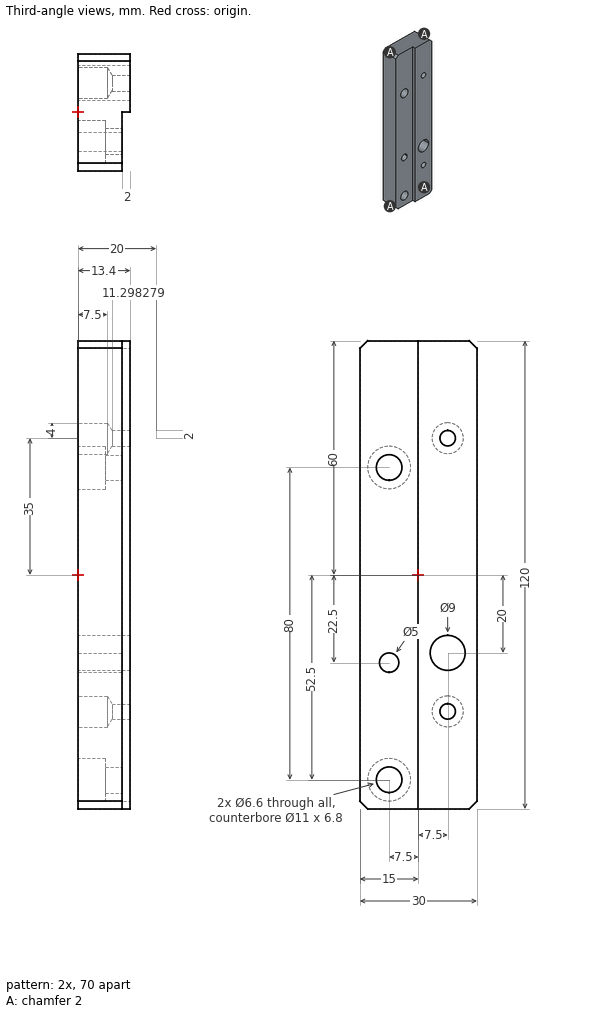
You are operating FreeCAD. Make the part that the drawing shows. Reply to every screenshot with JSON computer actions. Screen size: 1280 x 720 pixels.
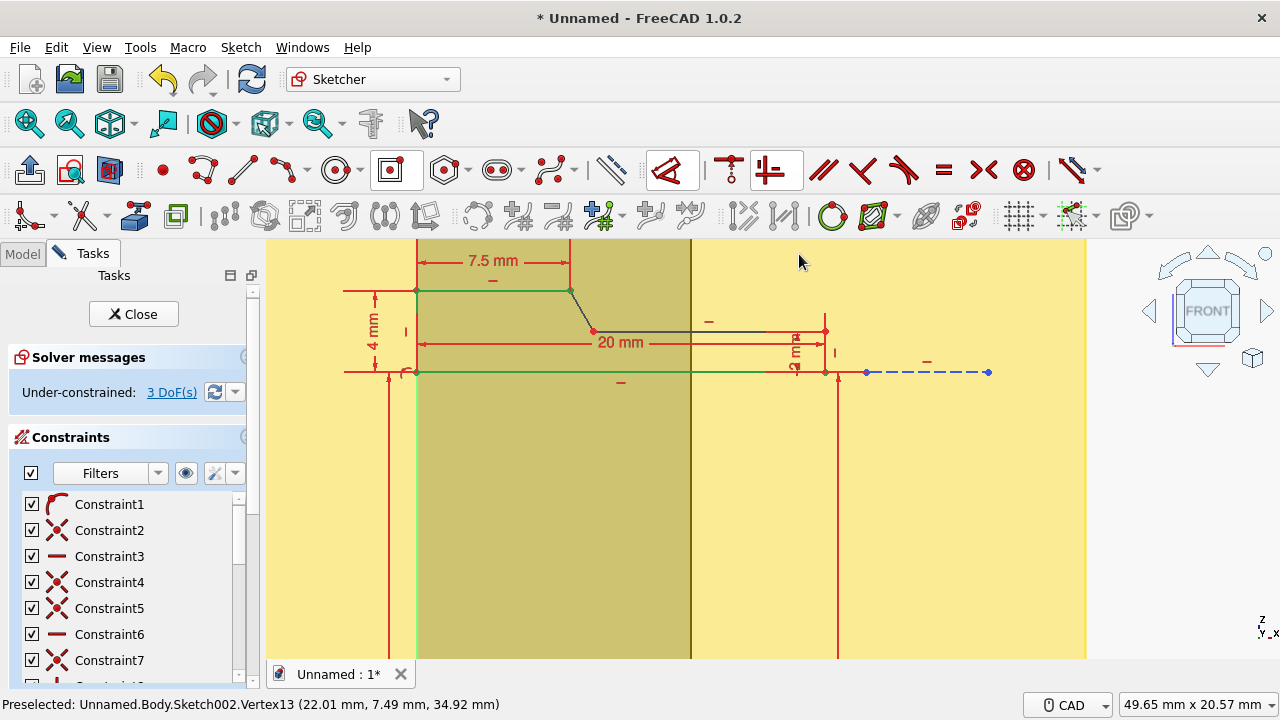
{"action": "left_click", "coordinate": [663, 332]}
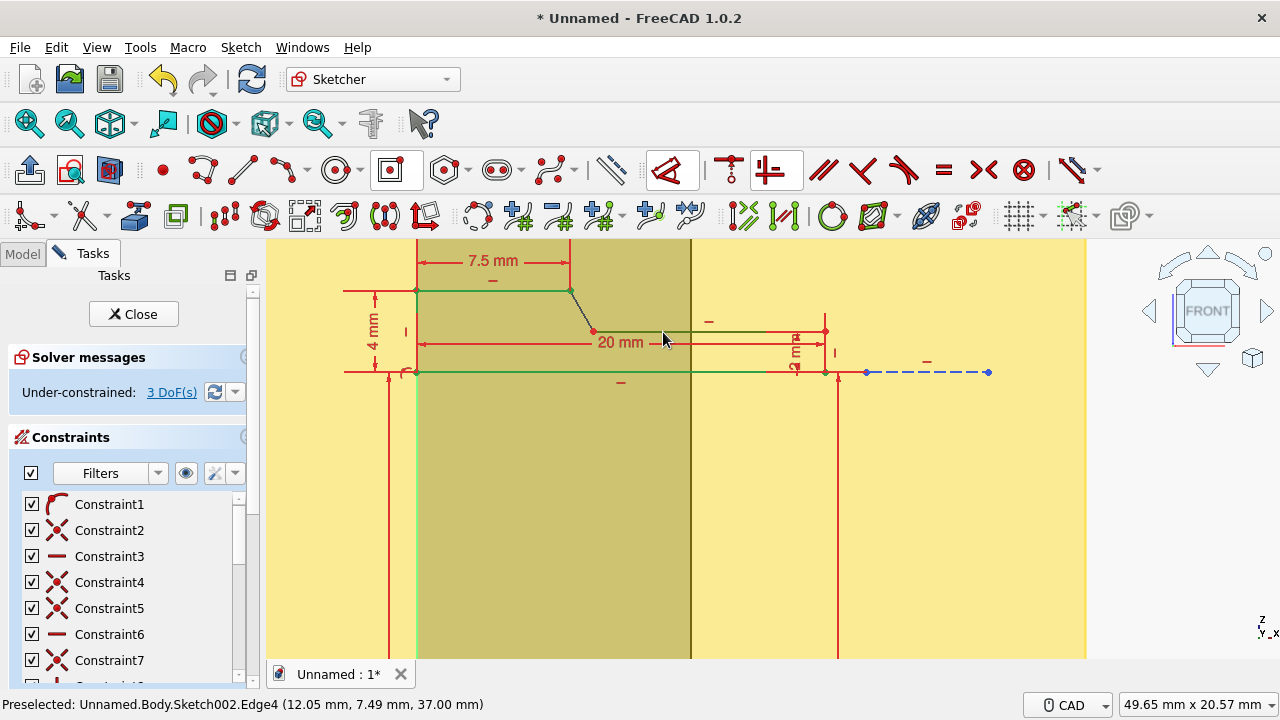
{"action": "left_click", "coordinate": [694, 170]}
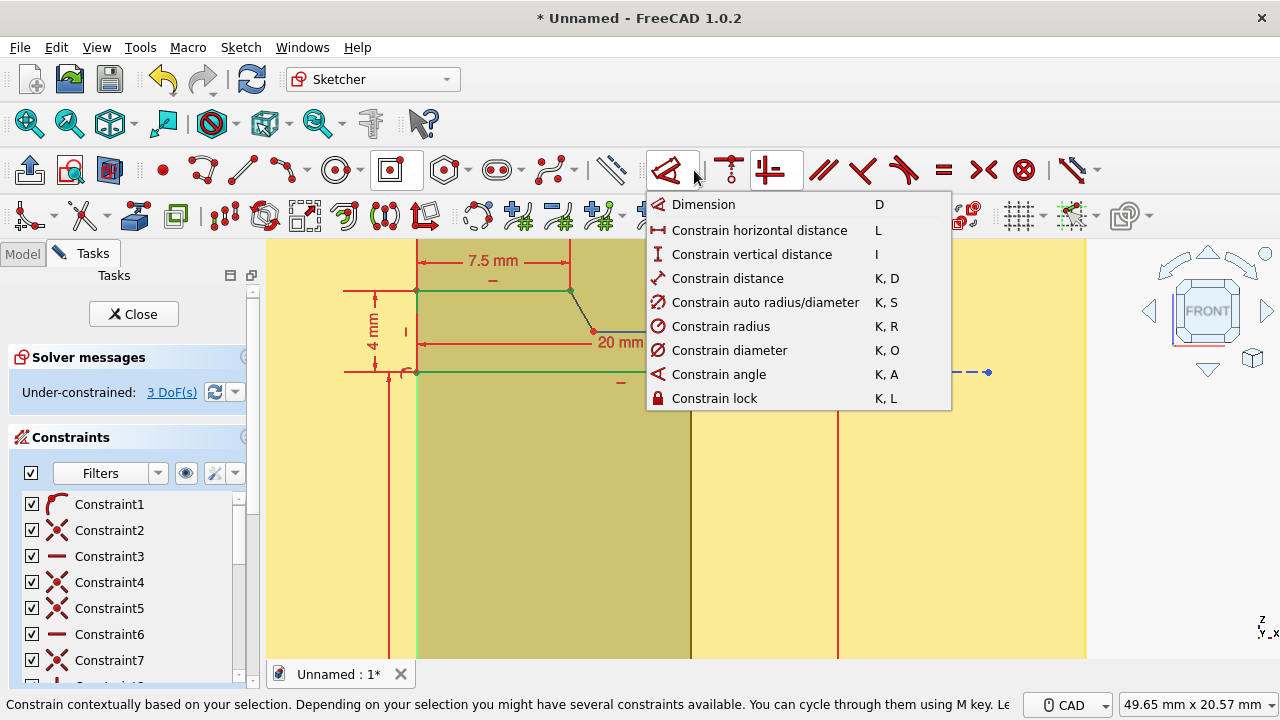
{"action": "left_click", "coordinate": [799, 230]}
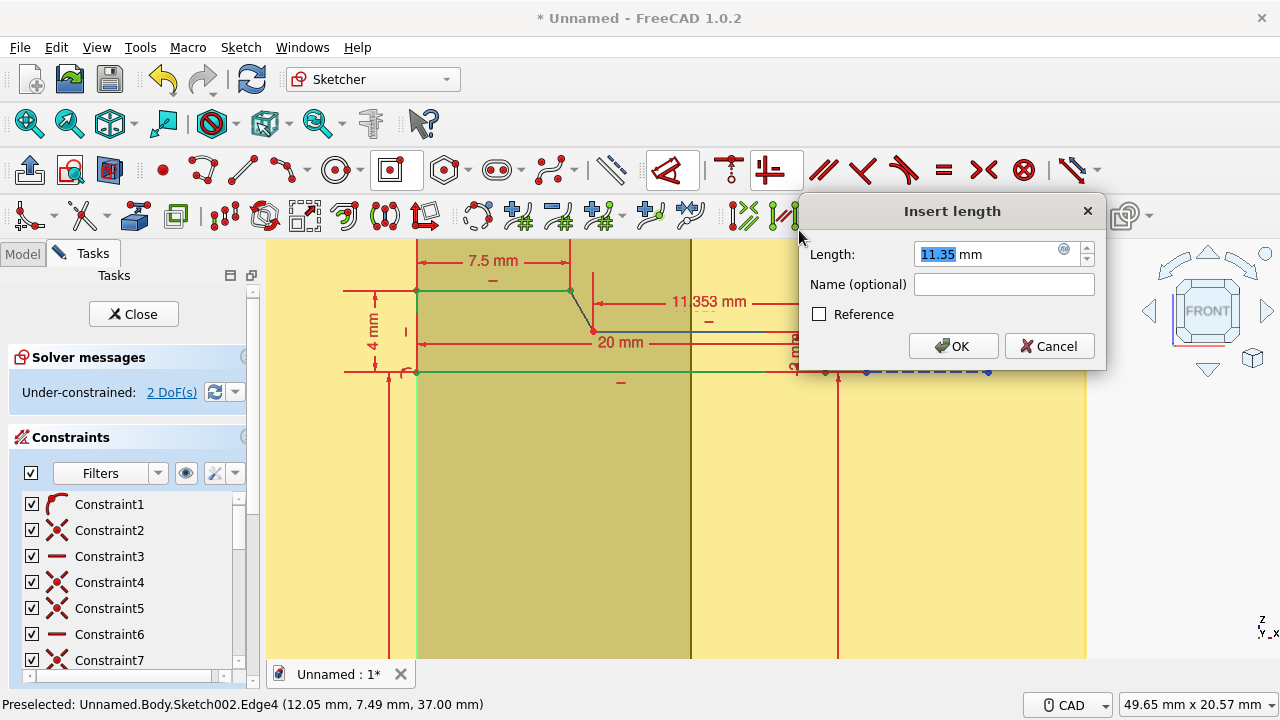
{"action": "type", "text": "11.298279"}
{"action": "key", "text": "Return"}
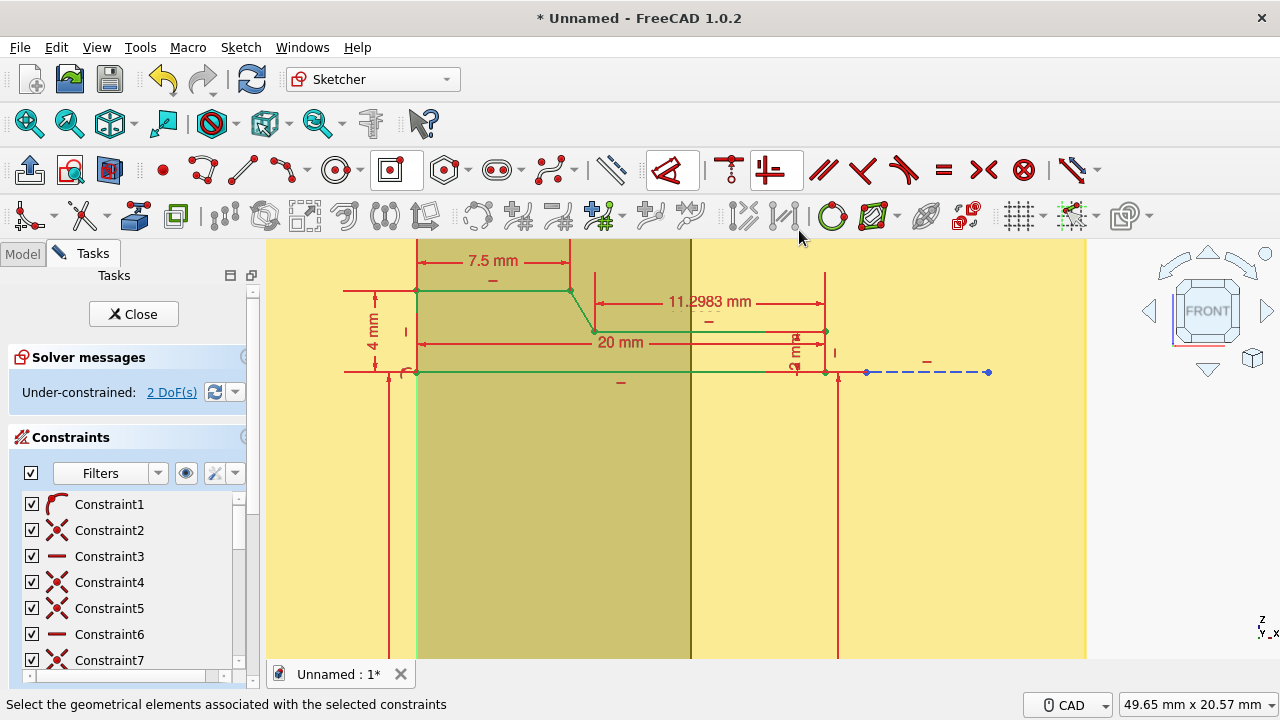
{"action": "left_click", "coordinate": [134, 314]}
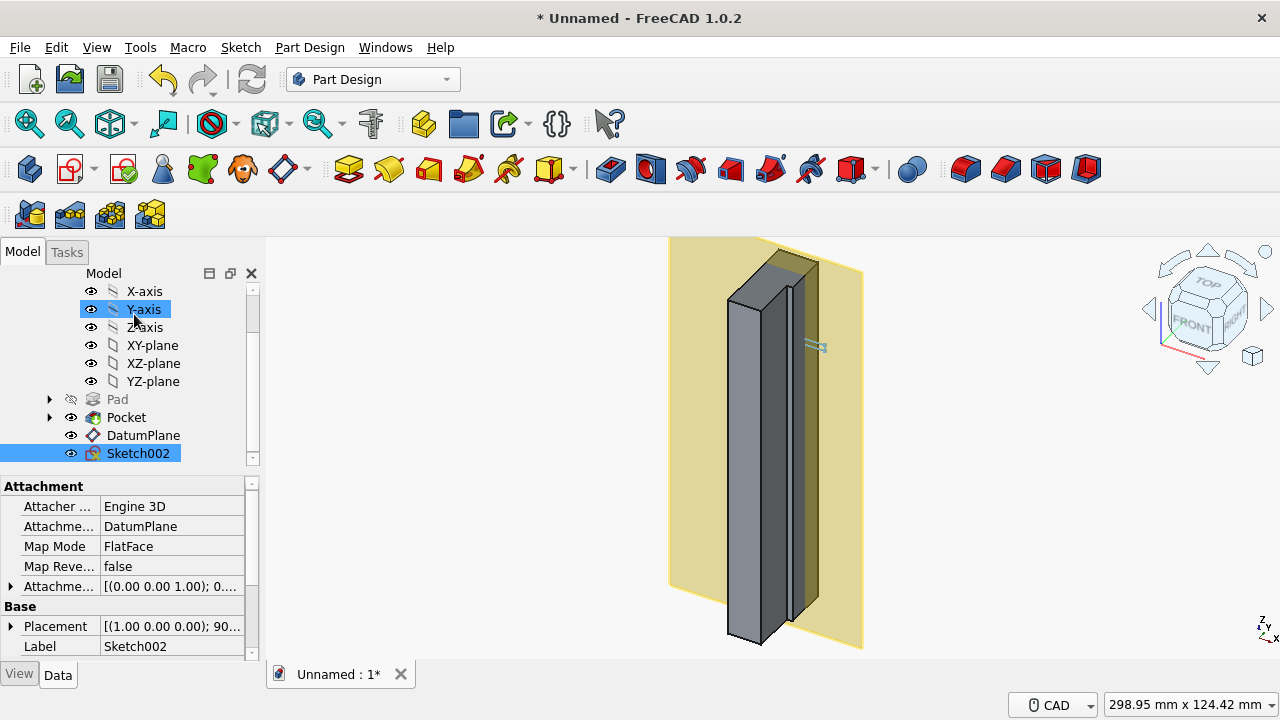
{"action": "left_click", "coordinate": [692, 170]}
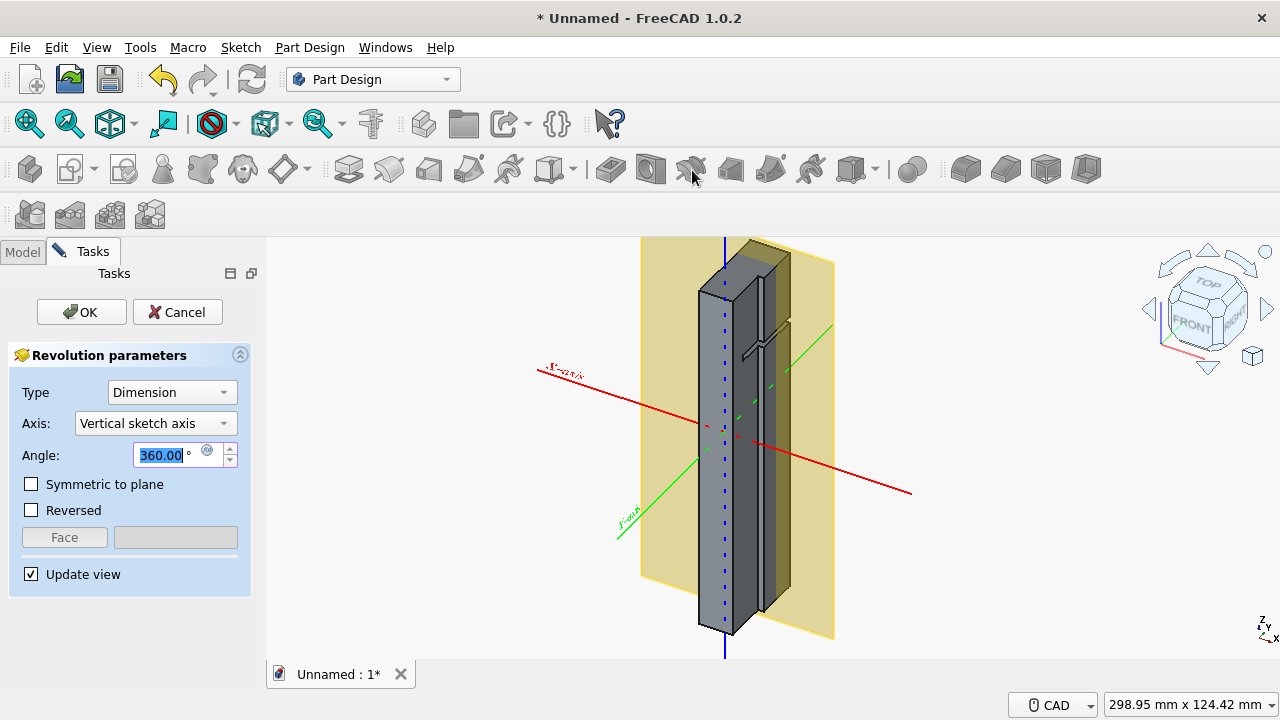
{"action": "left_click", "coordinate": [156, 424]}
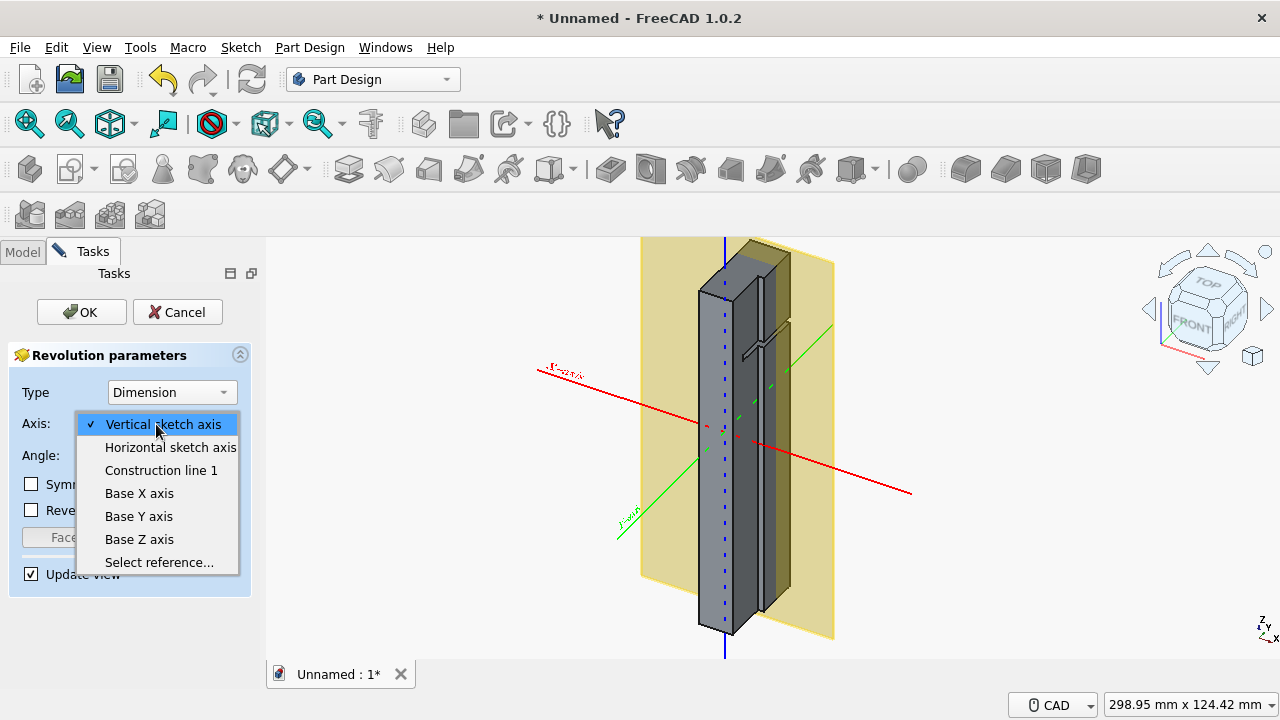
{"action": "left_click", "coordinate": [156, 470]}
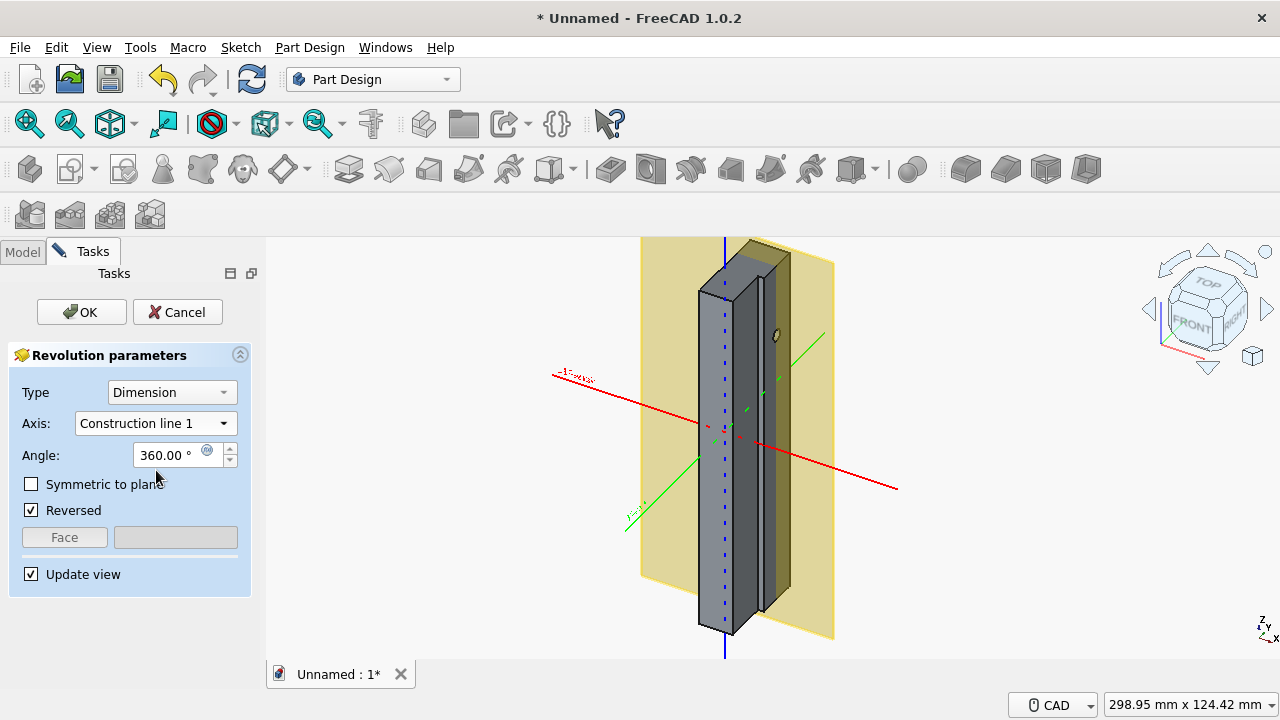
{"action": "left_click", "coordinate": [82, 312]}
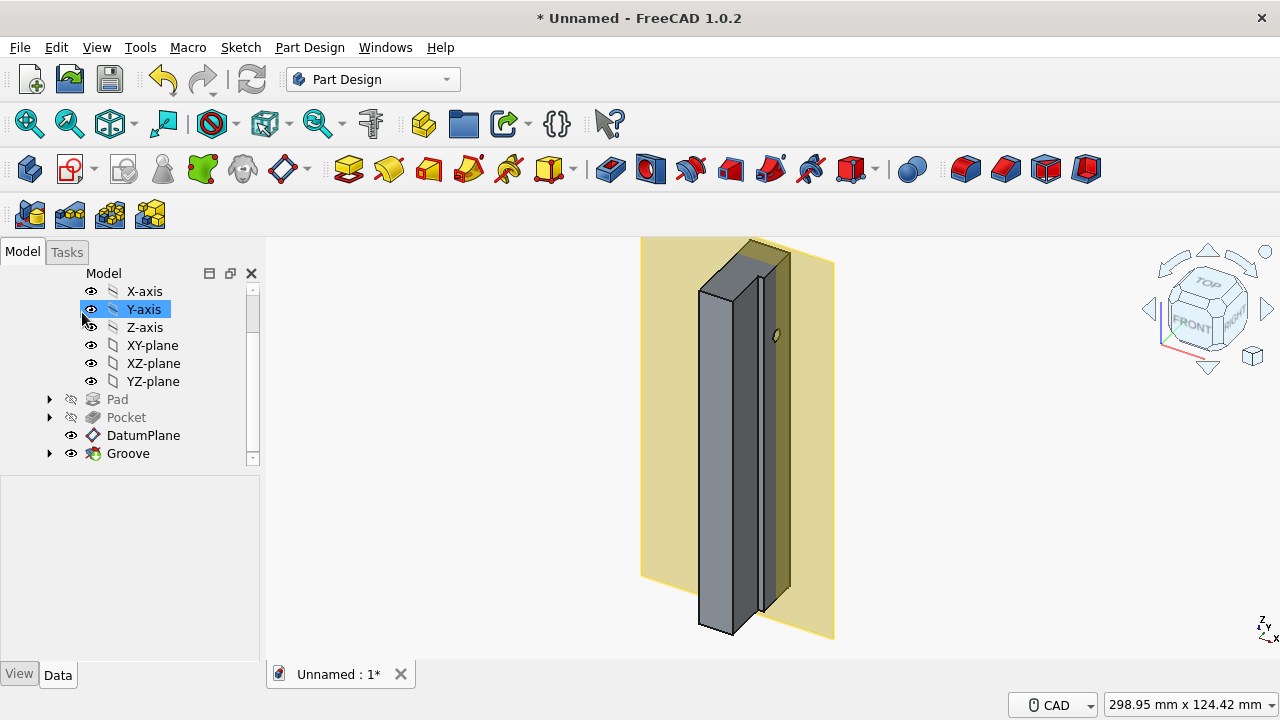
{"action": "left_click", "coordinate": [116, 435]}
{"action": "key", "text": "space"}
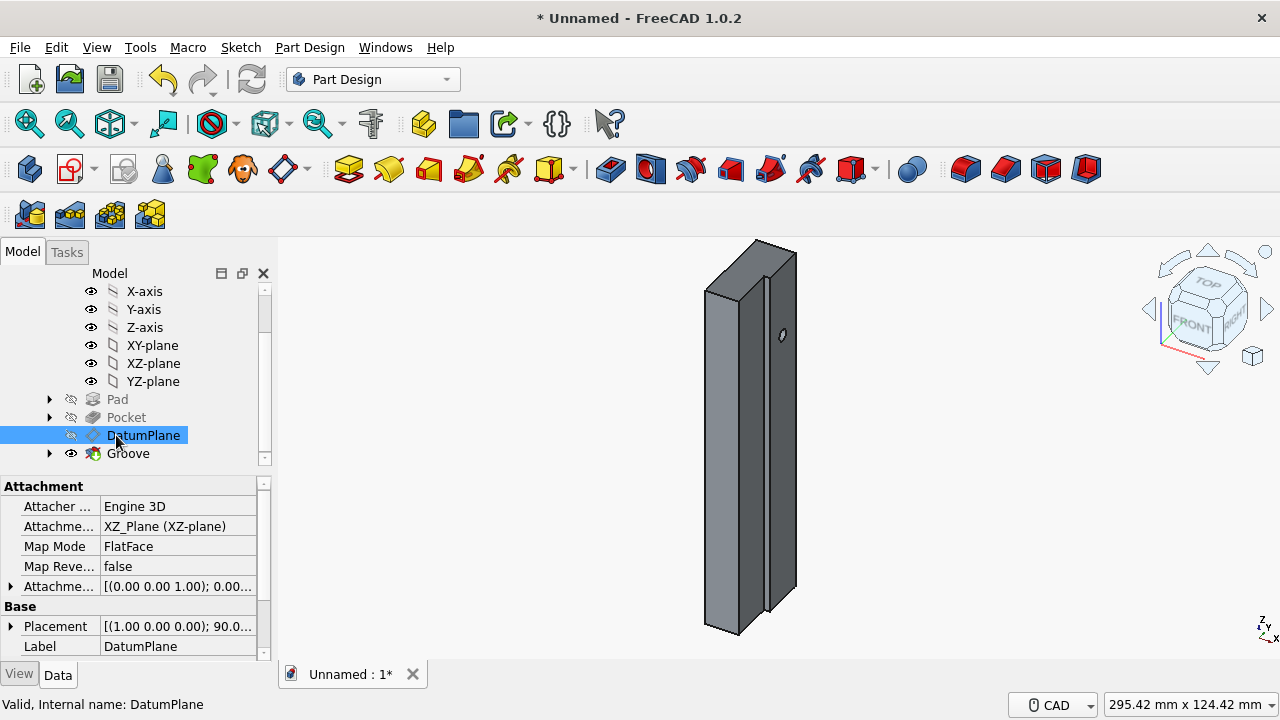
{"action": "left_click", "coordinate": [116, 453]}